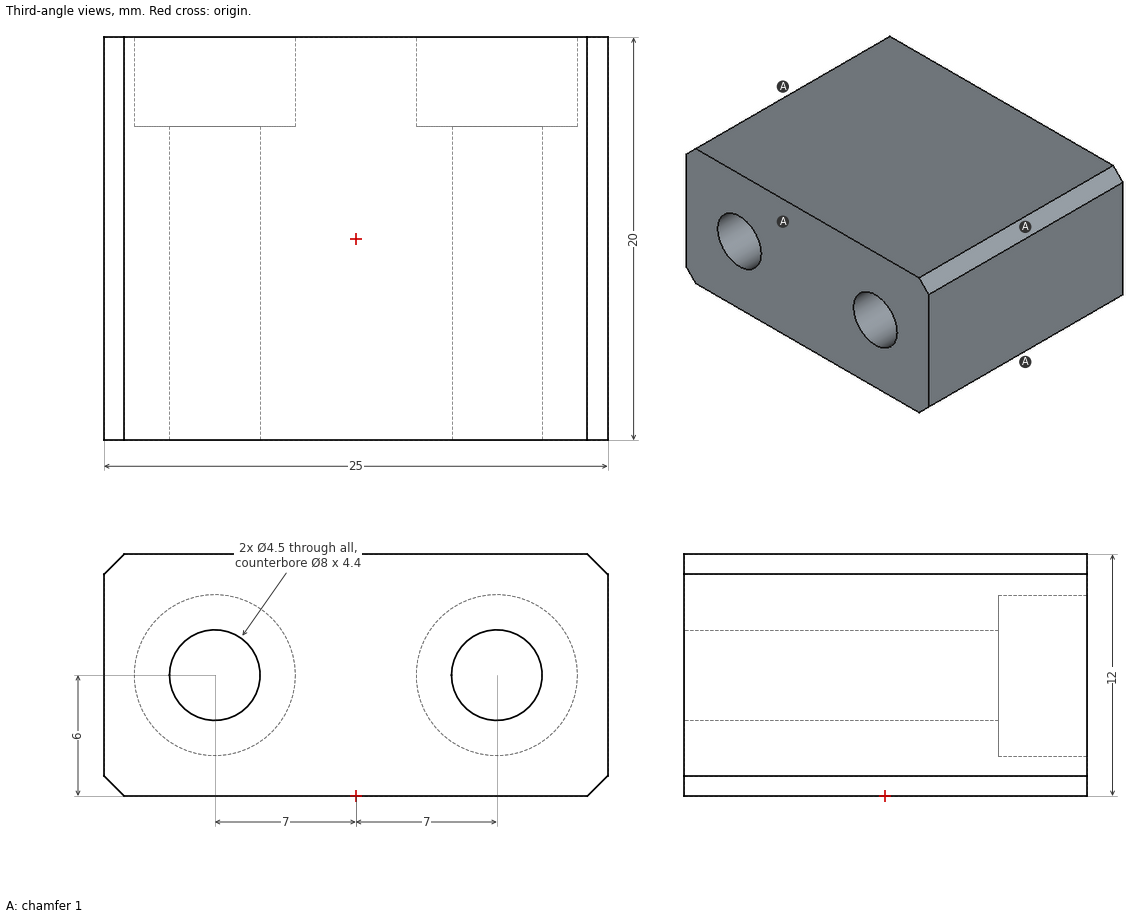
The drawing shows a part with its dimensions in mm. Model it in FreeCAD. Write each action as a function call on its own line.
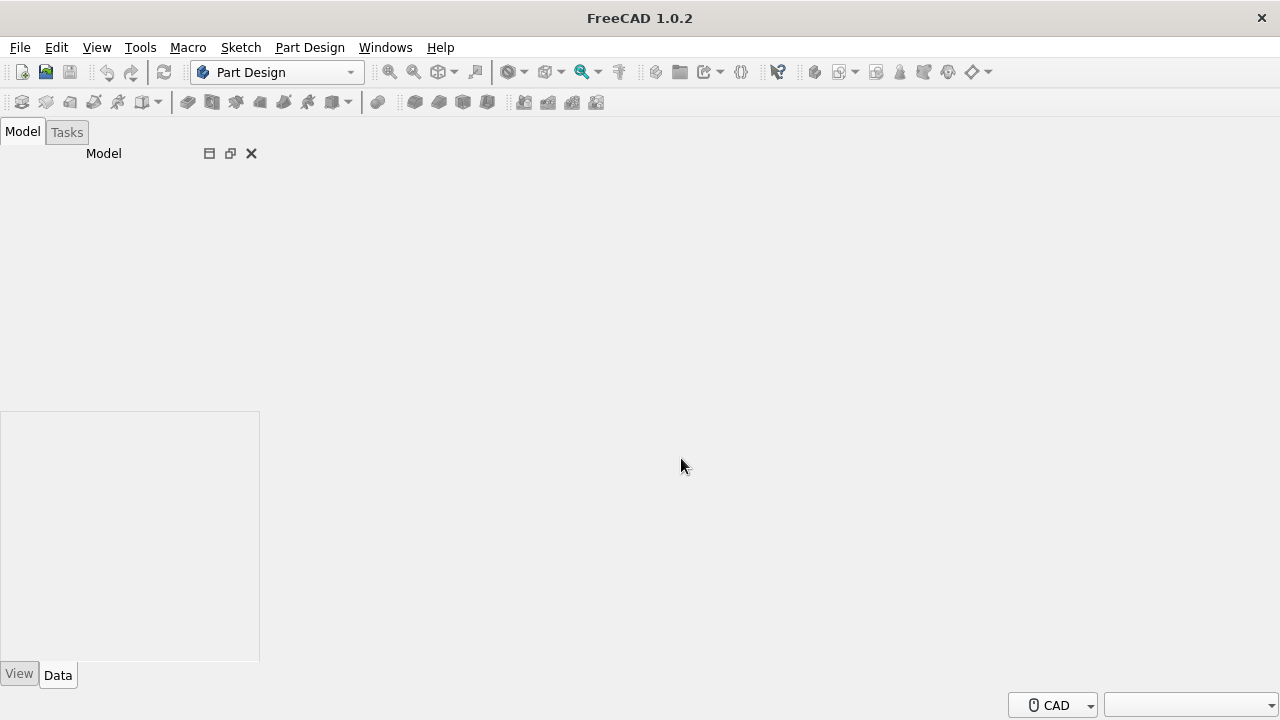
click(22, 72)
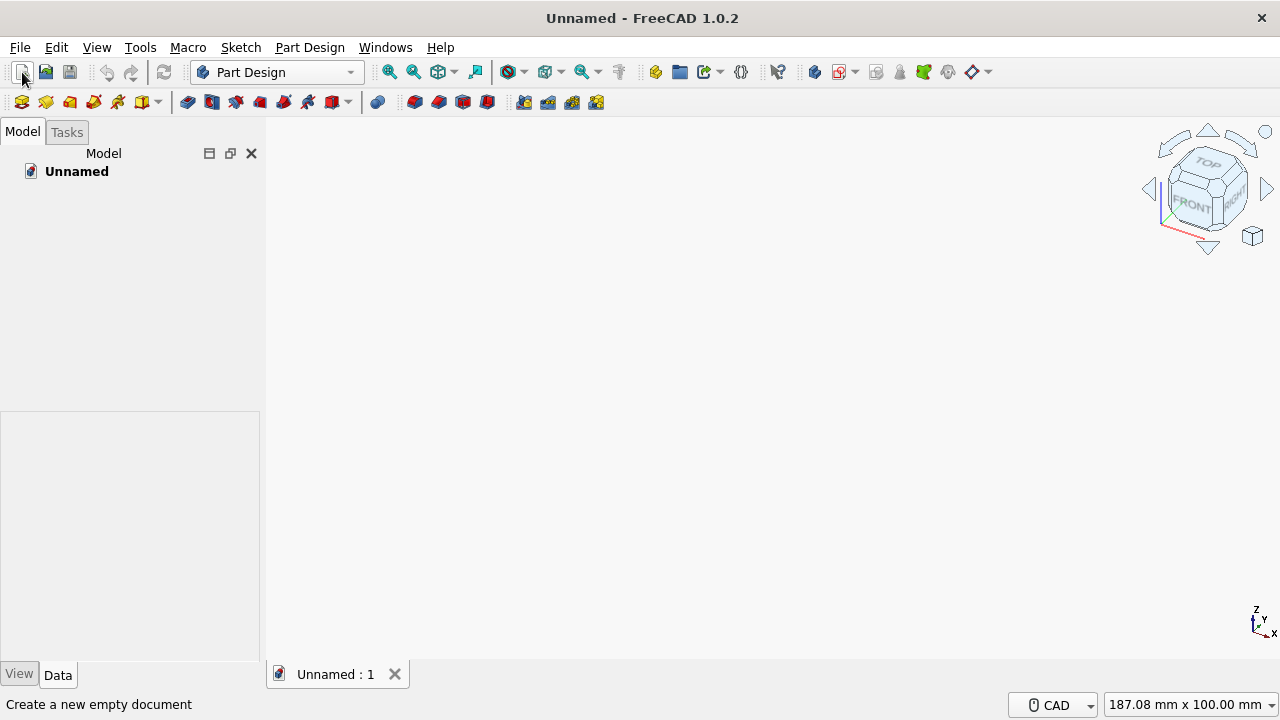
click(840, 72)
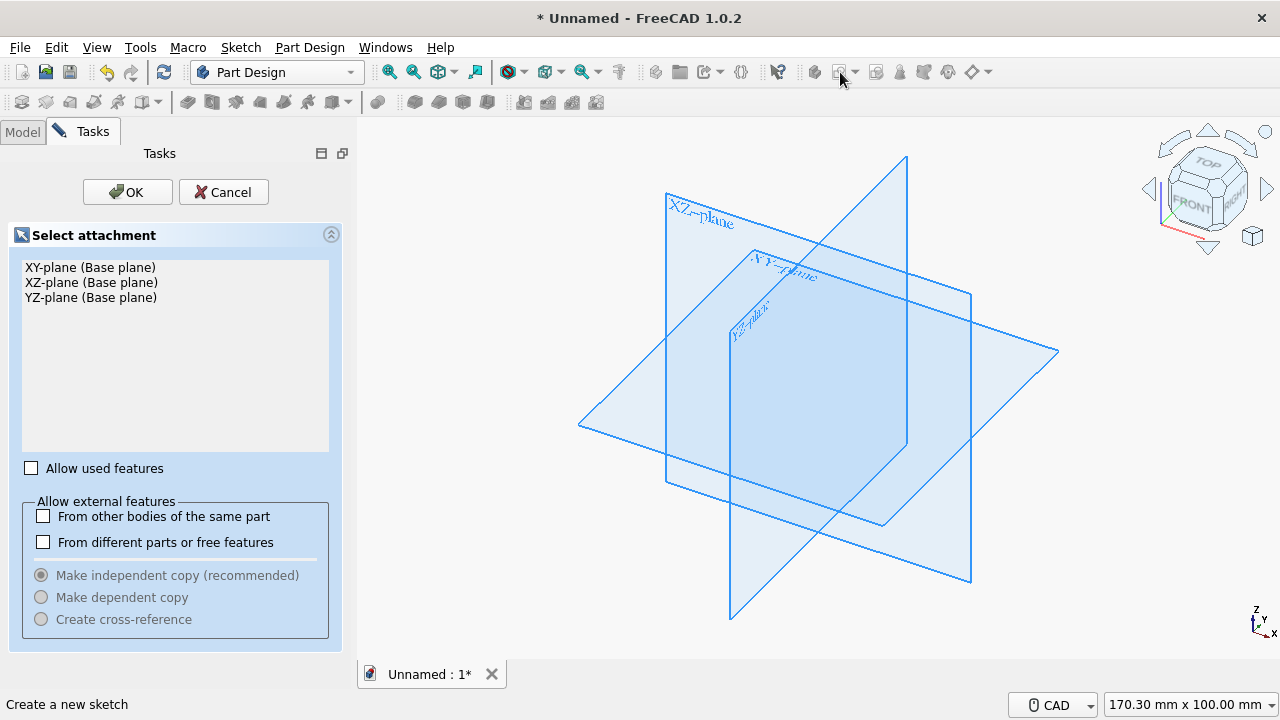
click(82, 268)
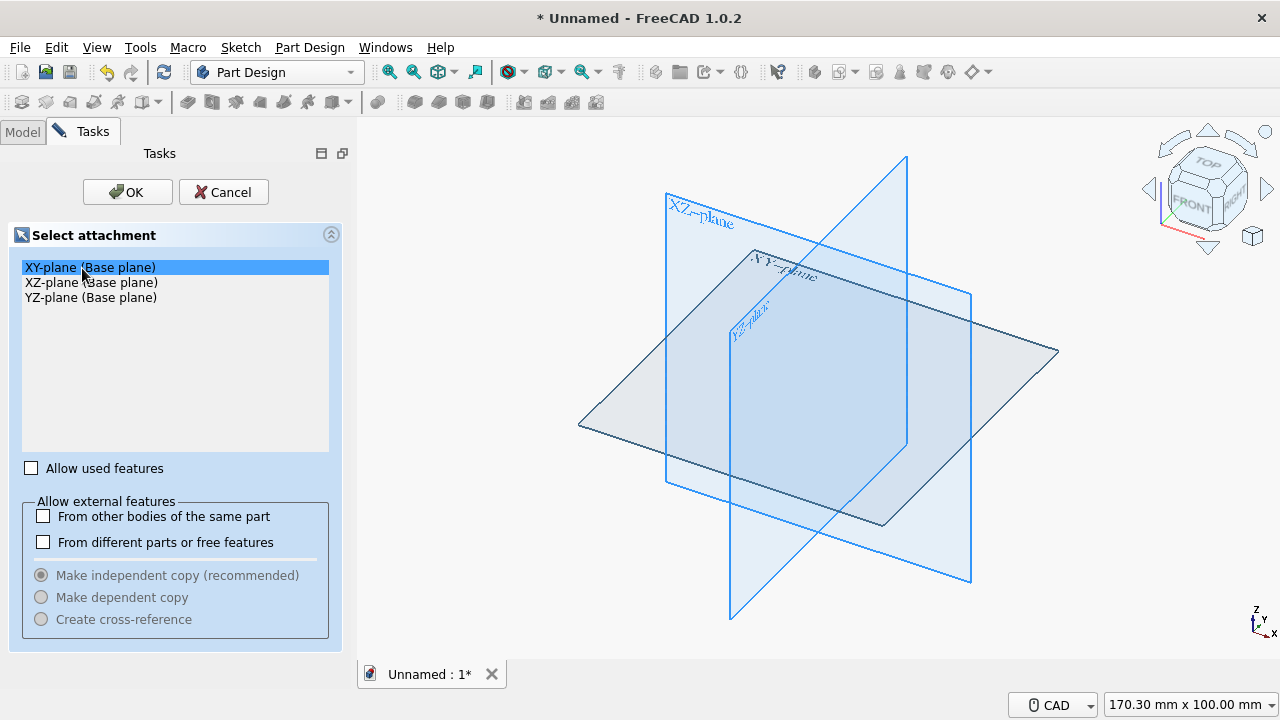
click(128, 192)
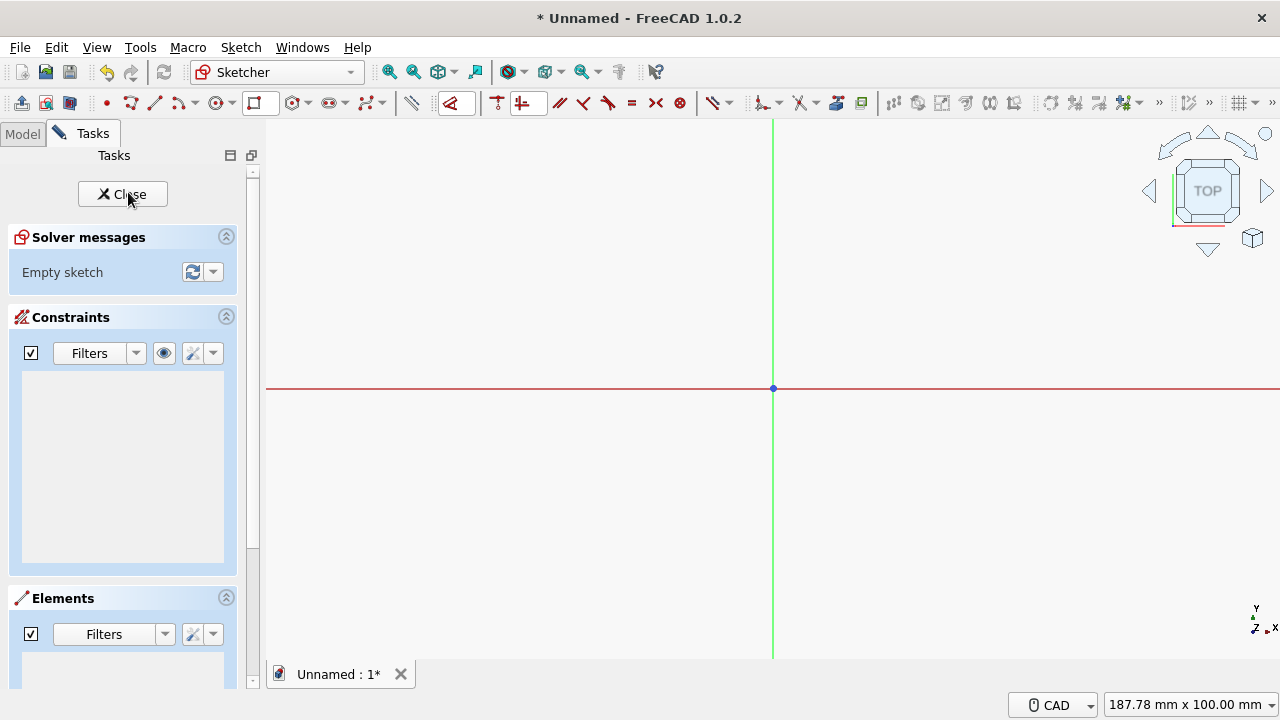
scroll(803, 389, up, 6)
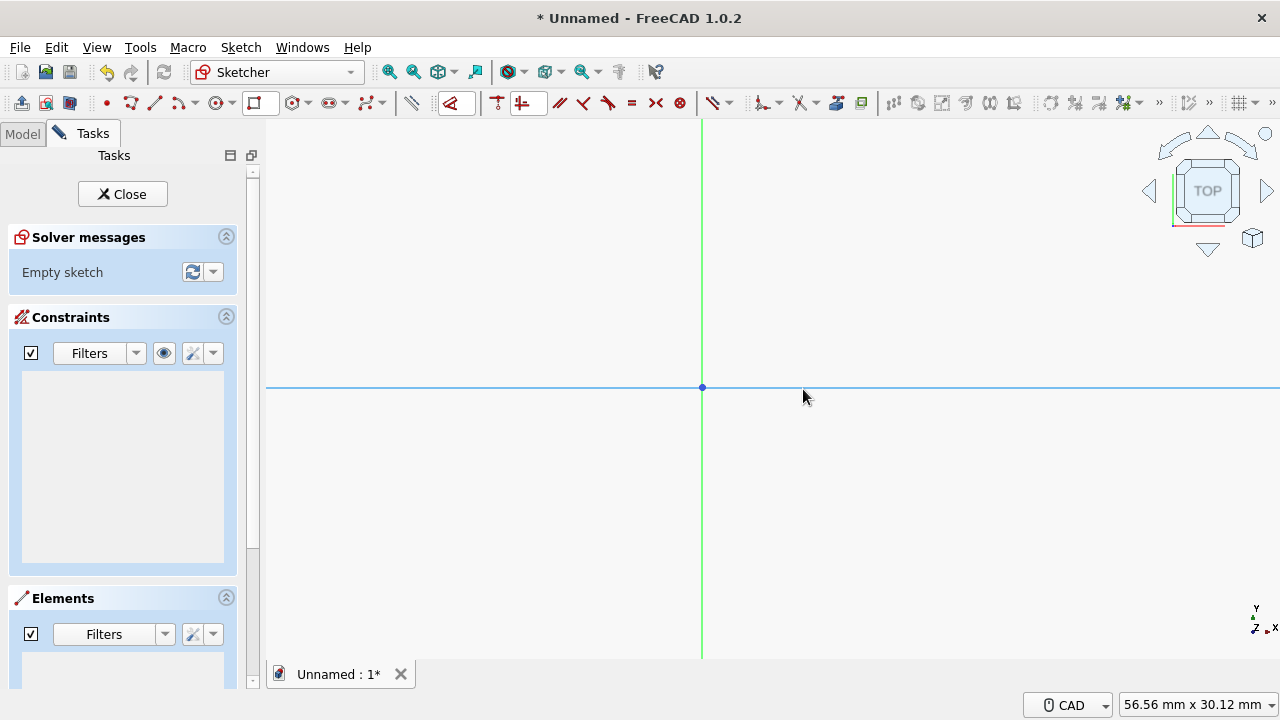
key(g)
key(v)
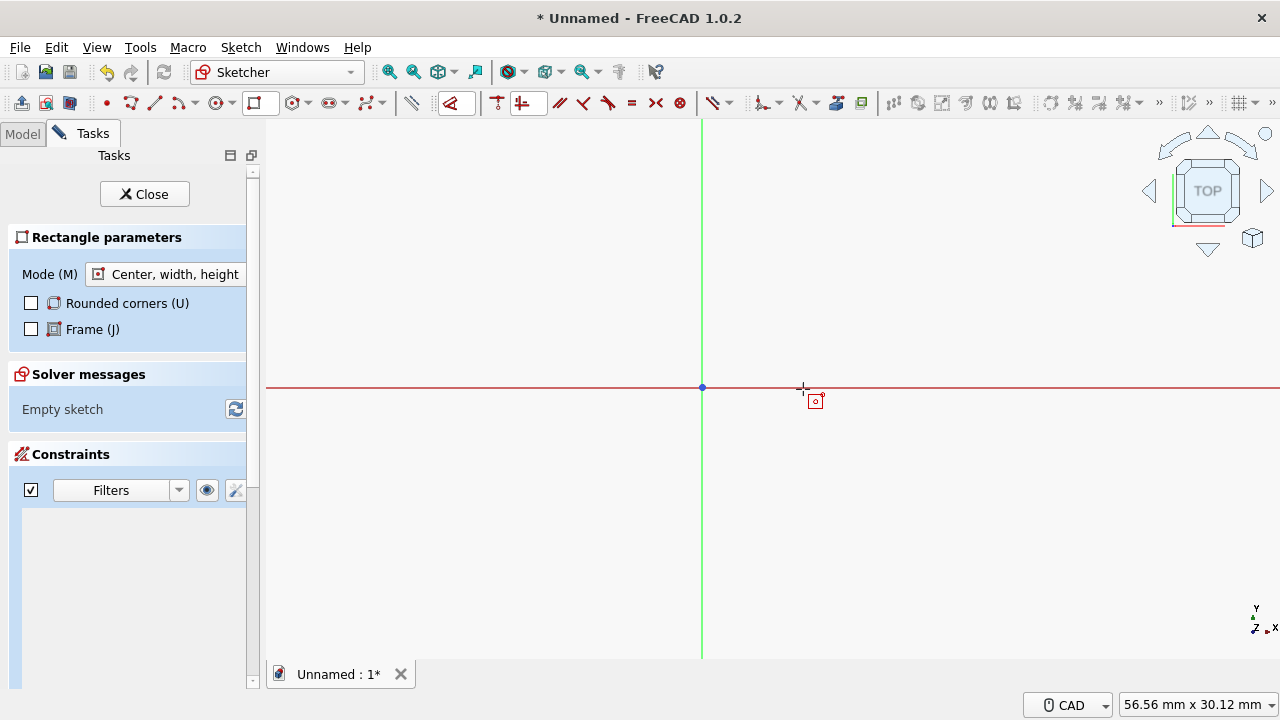
click(702, 388)
move(926, 209)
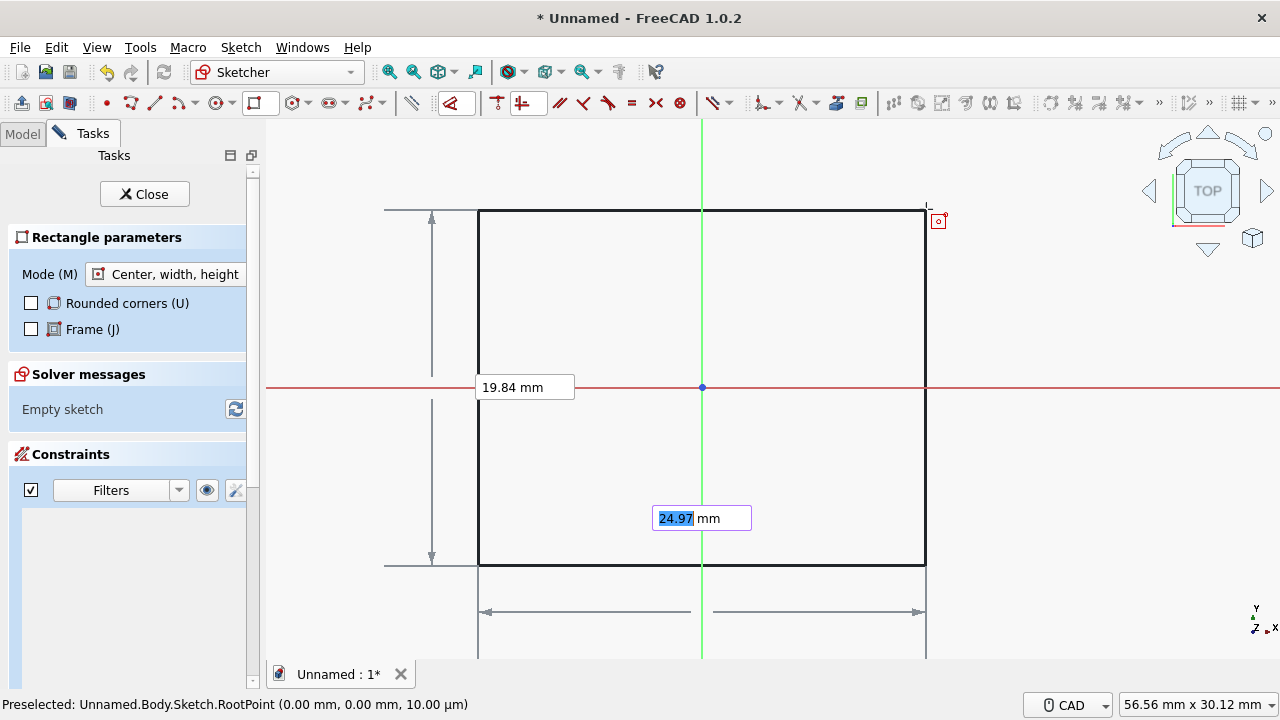
text(25)
key(Tab)
text(20)
key(Return)
key(Escape)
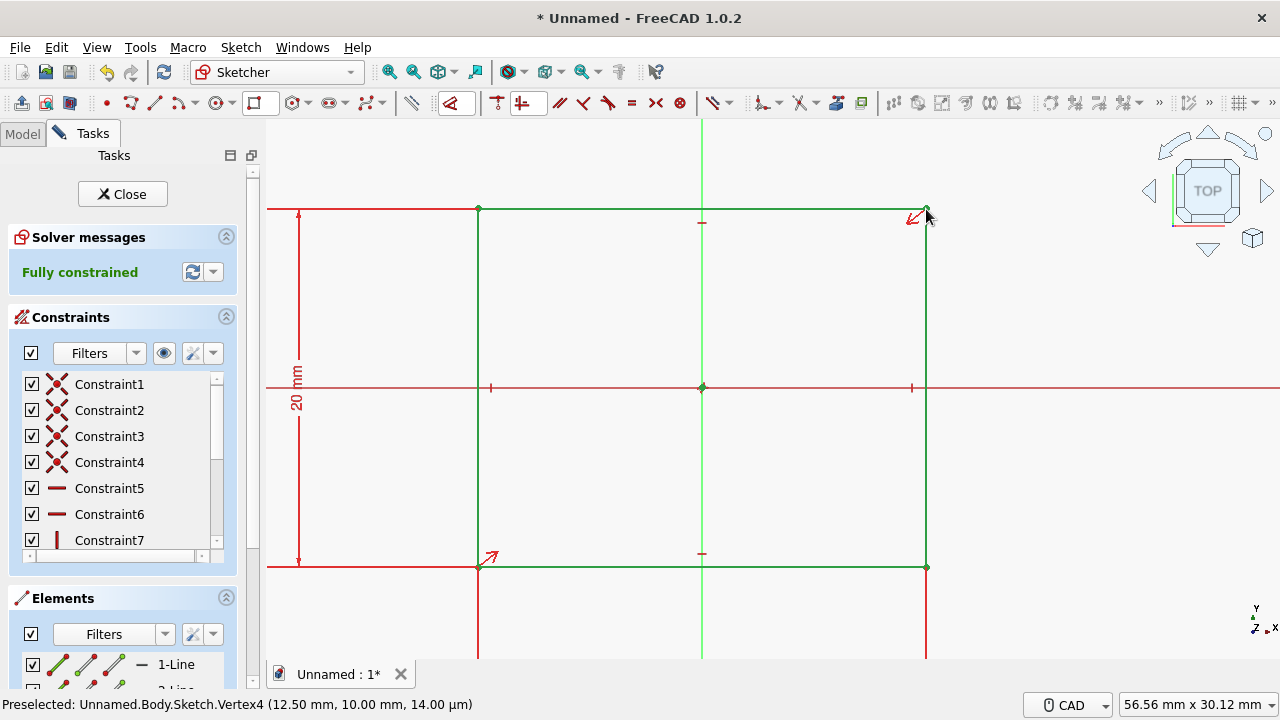
click(123, 194)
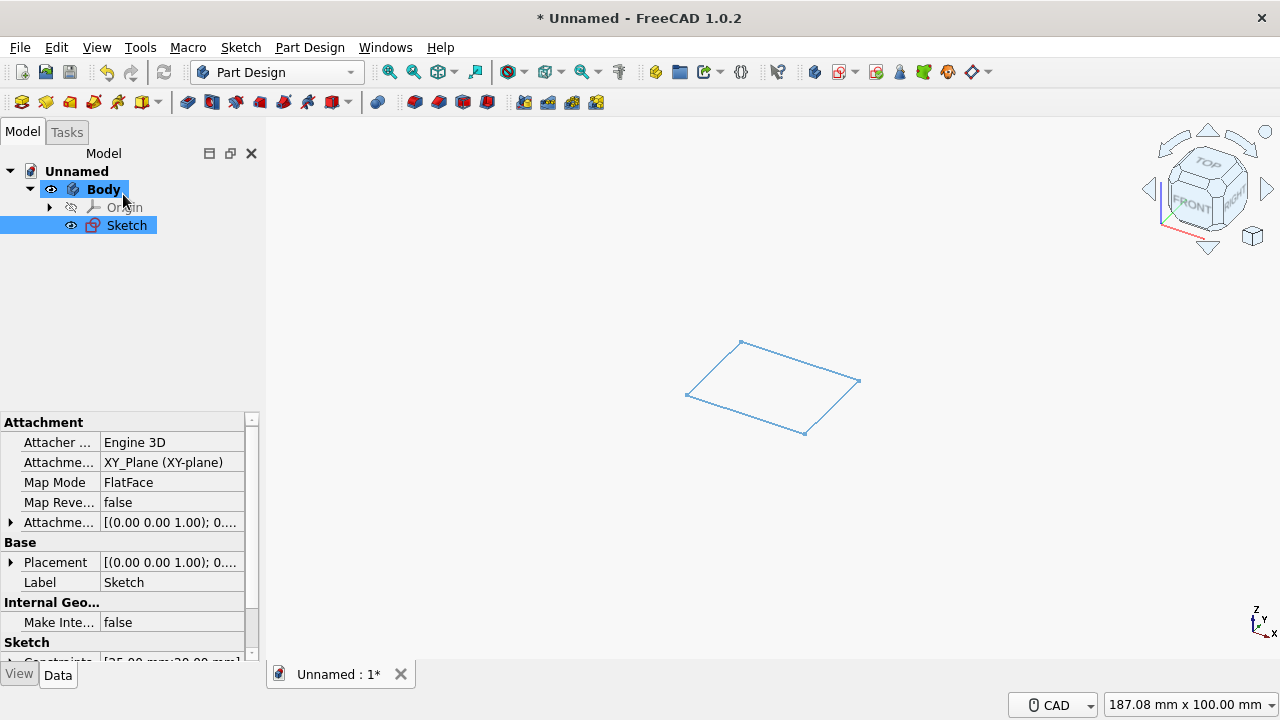
click(22, 102)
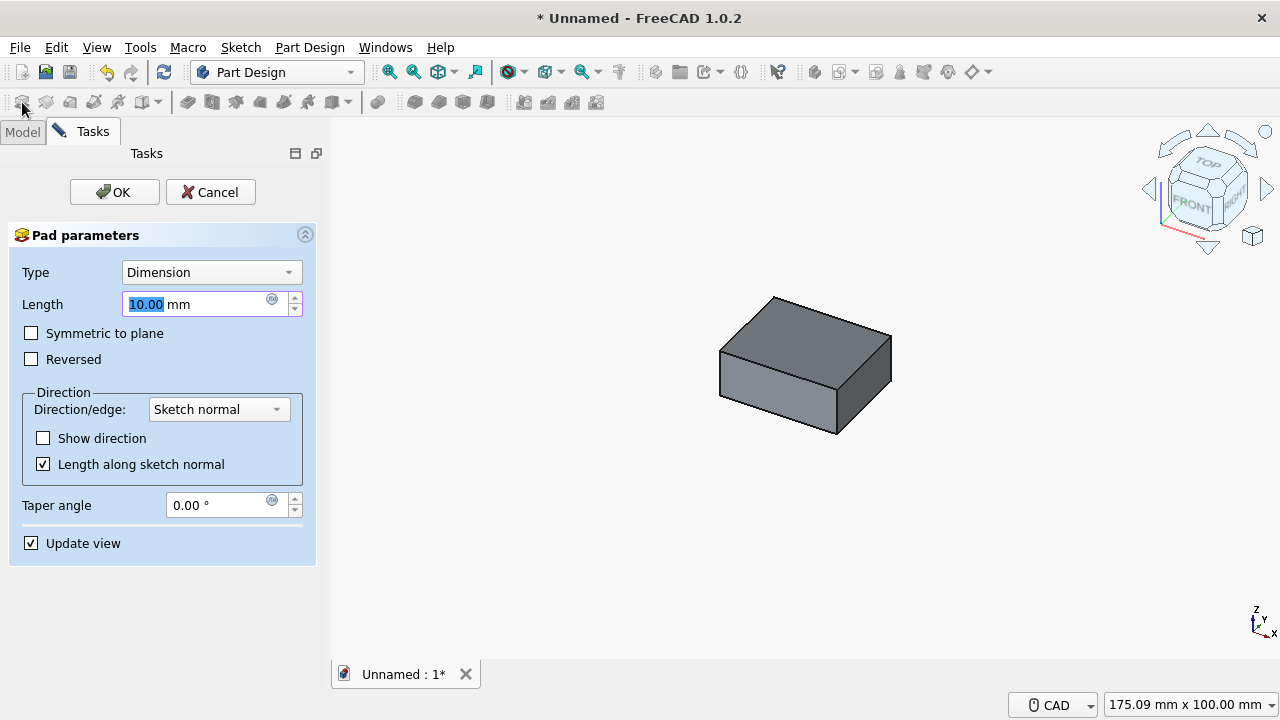
text(12)
key(Tab)